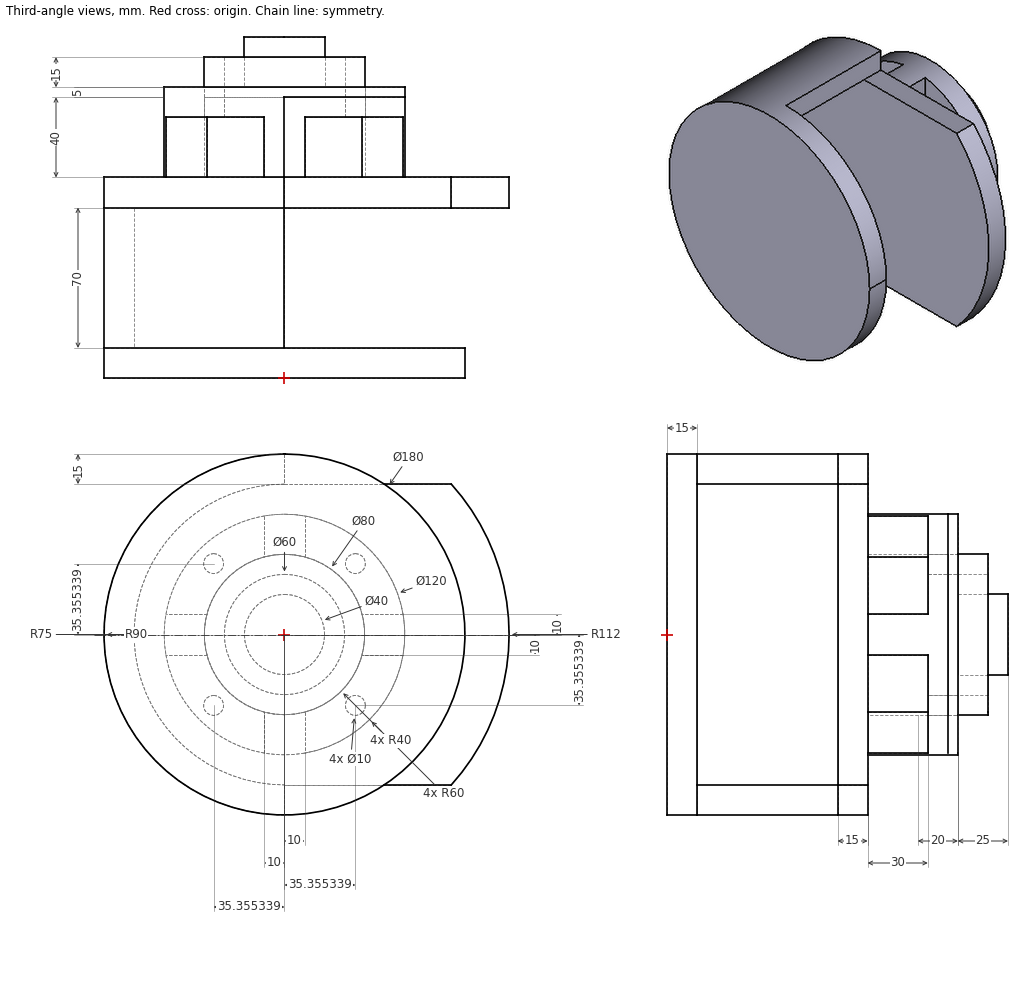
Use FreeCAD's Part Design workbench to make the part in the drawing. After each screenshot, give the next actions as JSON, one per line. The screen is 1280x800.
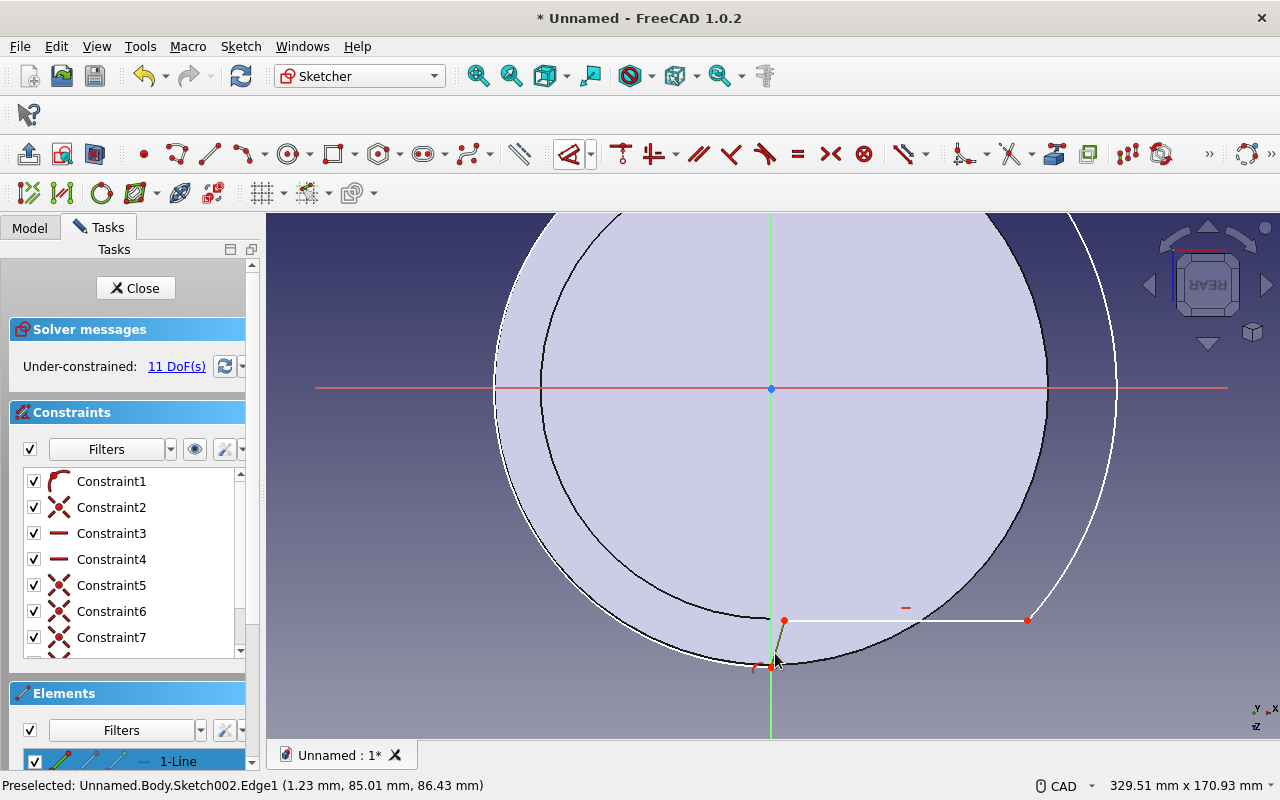
{"action": "left_click", "coordinate": [676, 154]}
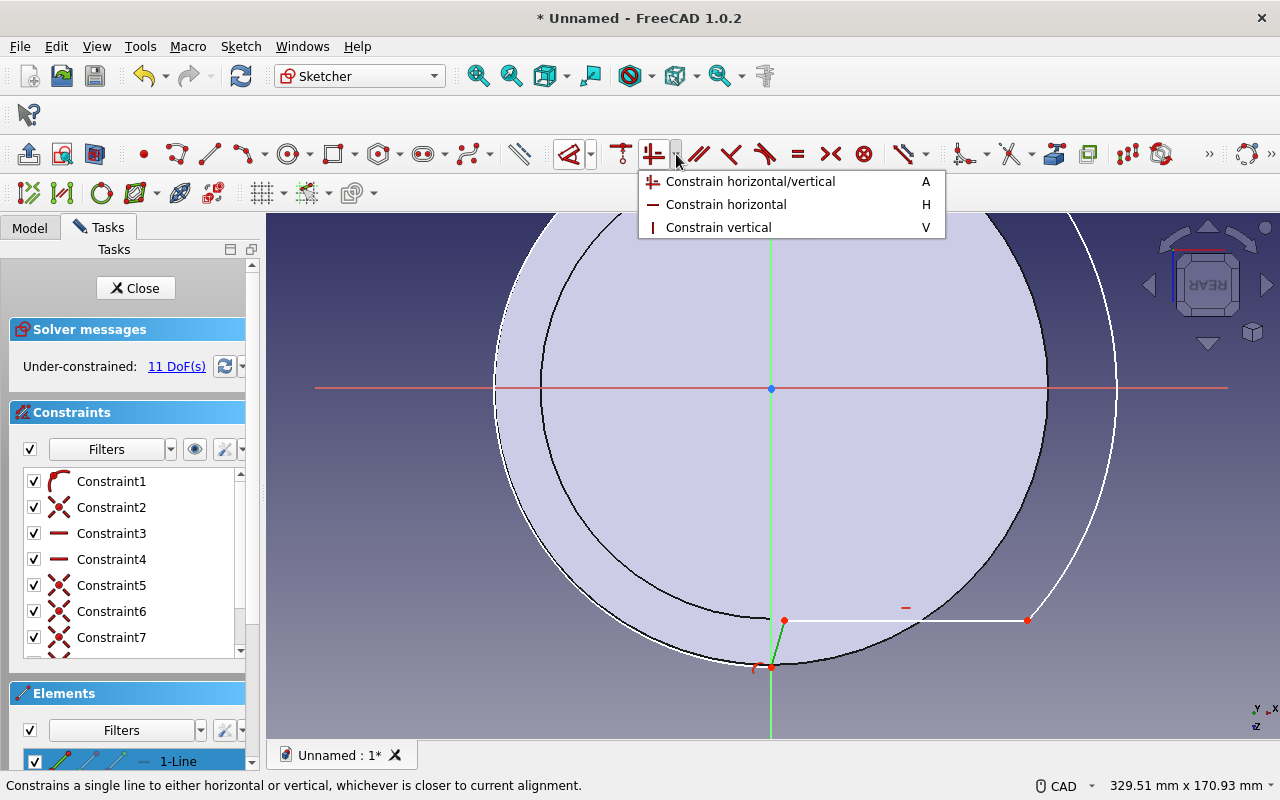
{"action": "left_click", "coordinate": [792, 228]}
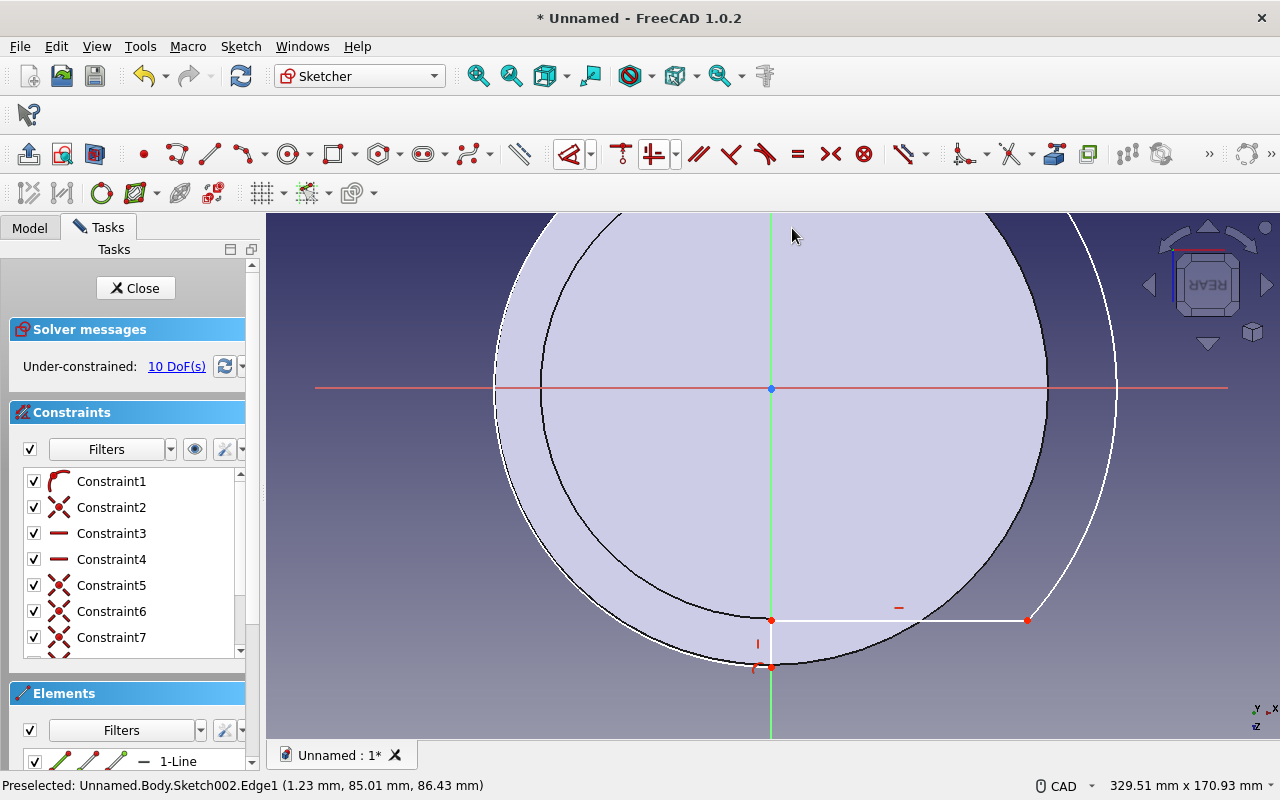
{"action": "scroll", "coordinate": [582, 583], "scroll_direction": "down", "scroll_amount": 3}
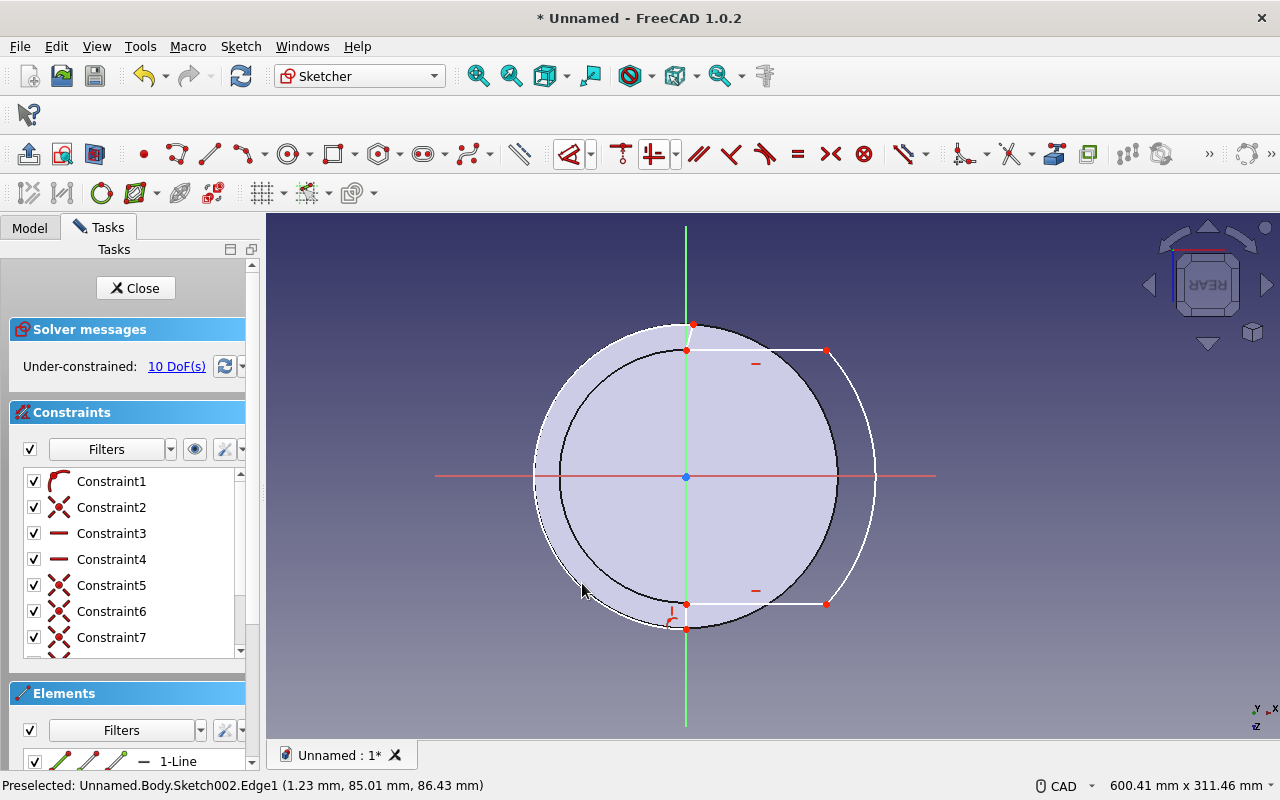
{"action": "scroll", "coordinate": [691, 332], "scroll_direction": "up", "scroll_amount": 5}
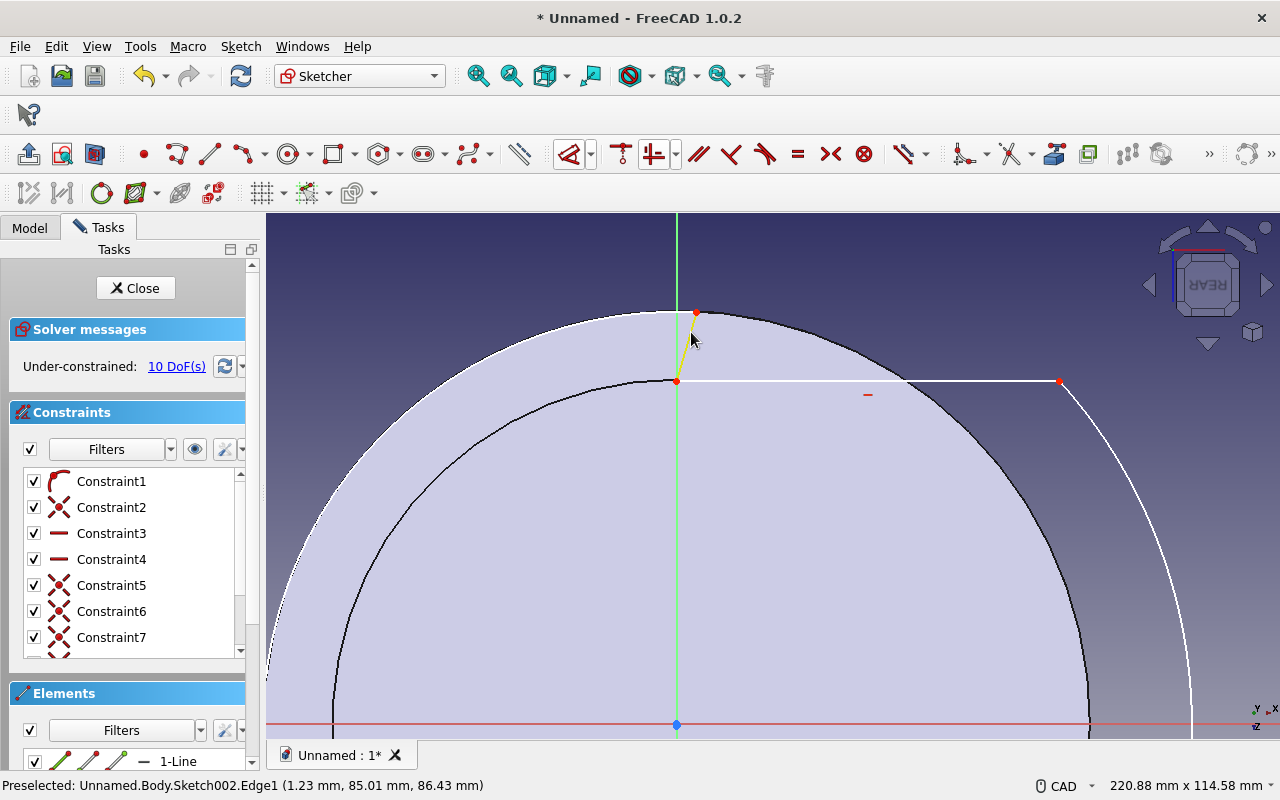
{"action": "left_click", "coordinate": [691, 333]}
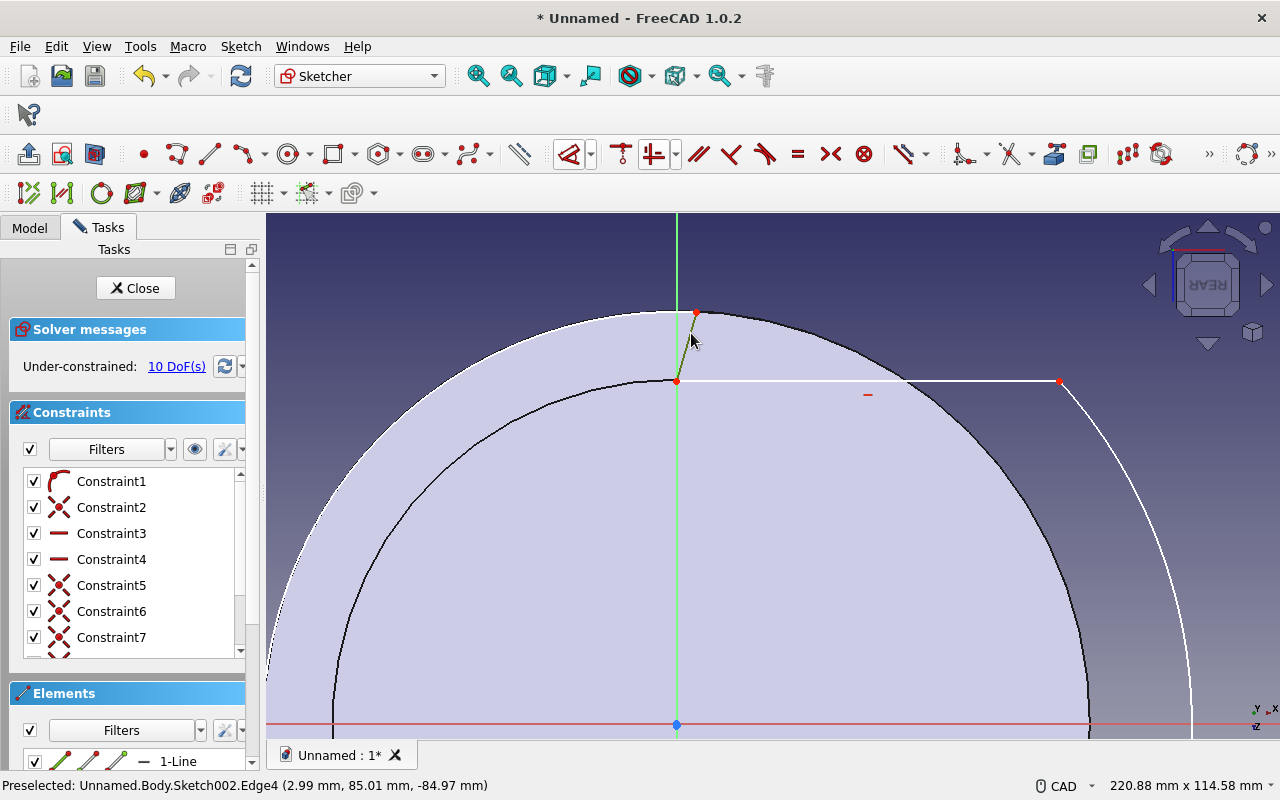
{"action": "left_click", "coordinate": [676, 154]}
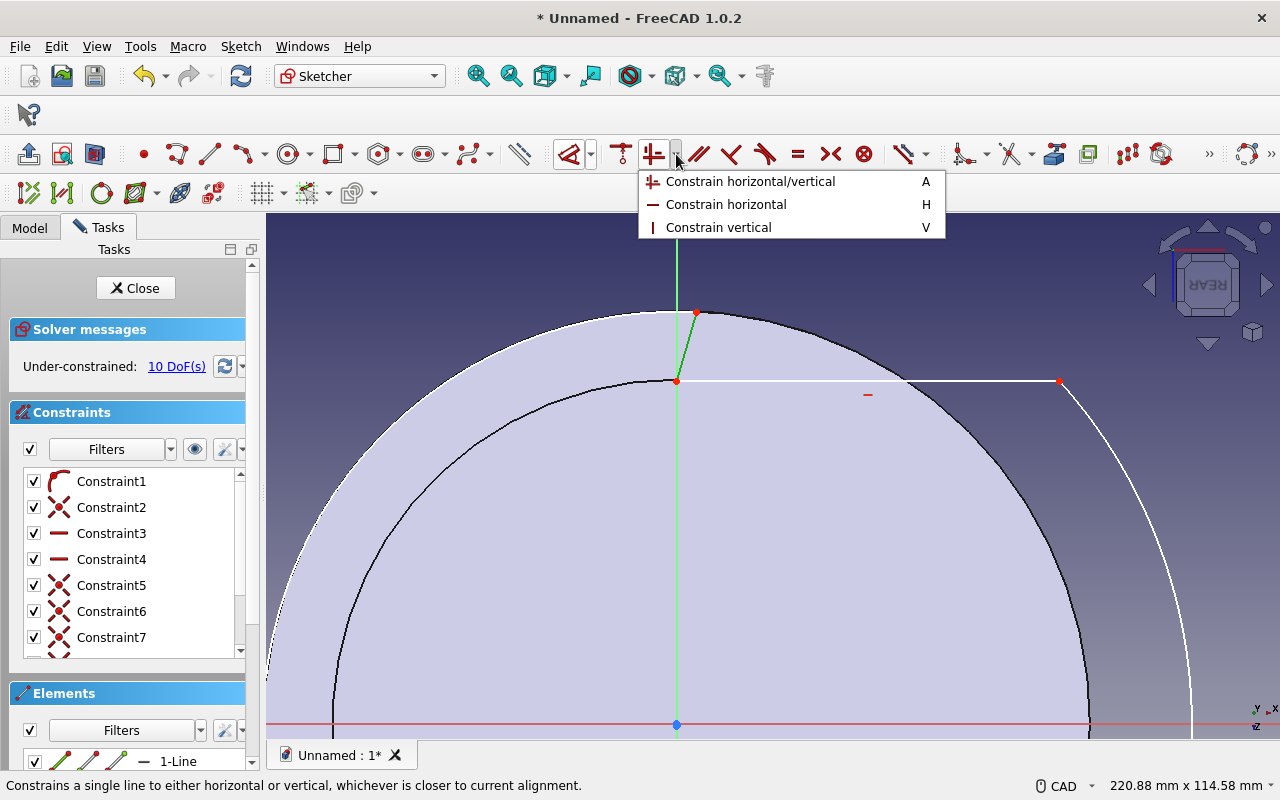
{"action": "left_click", "coordinate": [792, 228]}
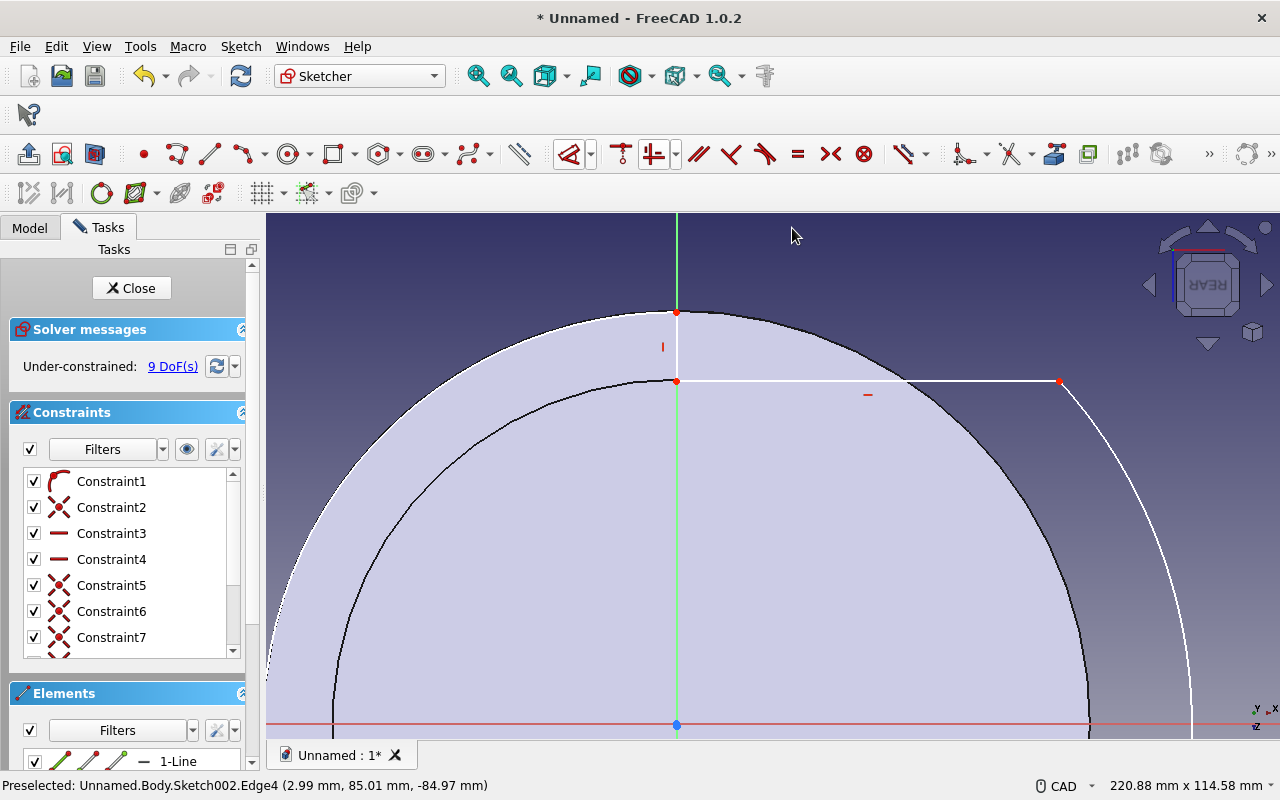
{"action": "scroll", "coordinate": [691, 332], "scroll_direction": "down", "scroll_amount": 5}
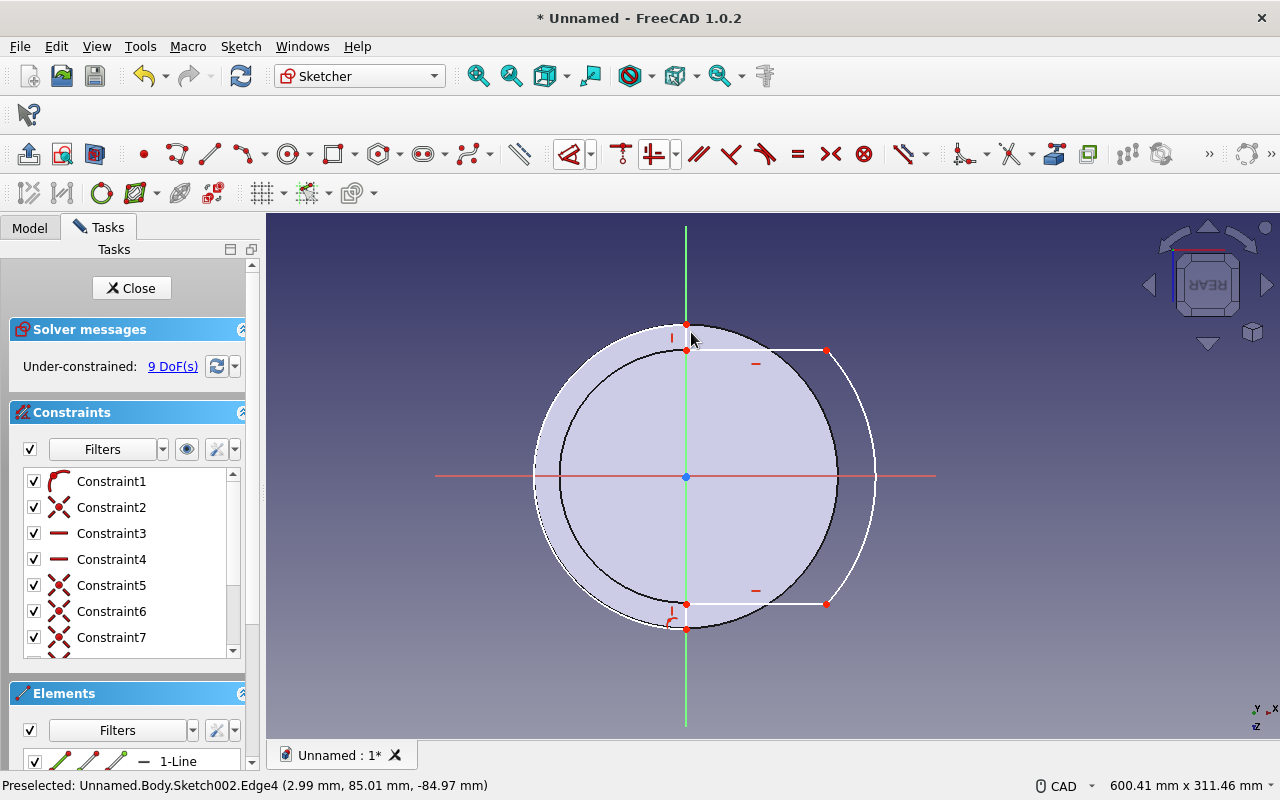
{"action": "left_click", "coordinate": [867, 532]}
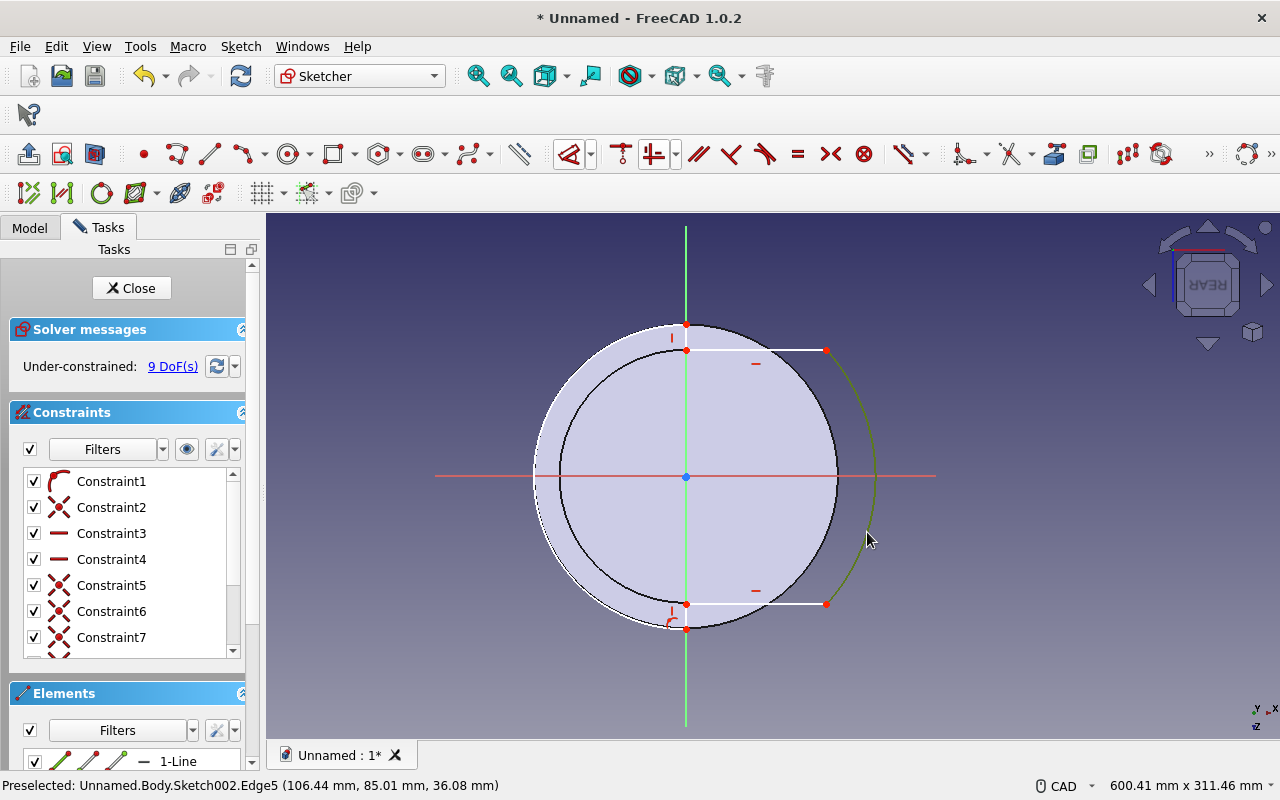
{"action": "left_click", "coordinate": [563, 388]}